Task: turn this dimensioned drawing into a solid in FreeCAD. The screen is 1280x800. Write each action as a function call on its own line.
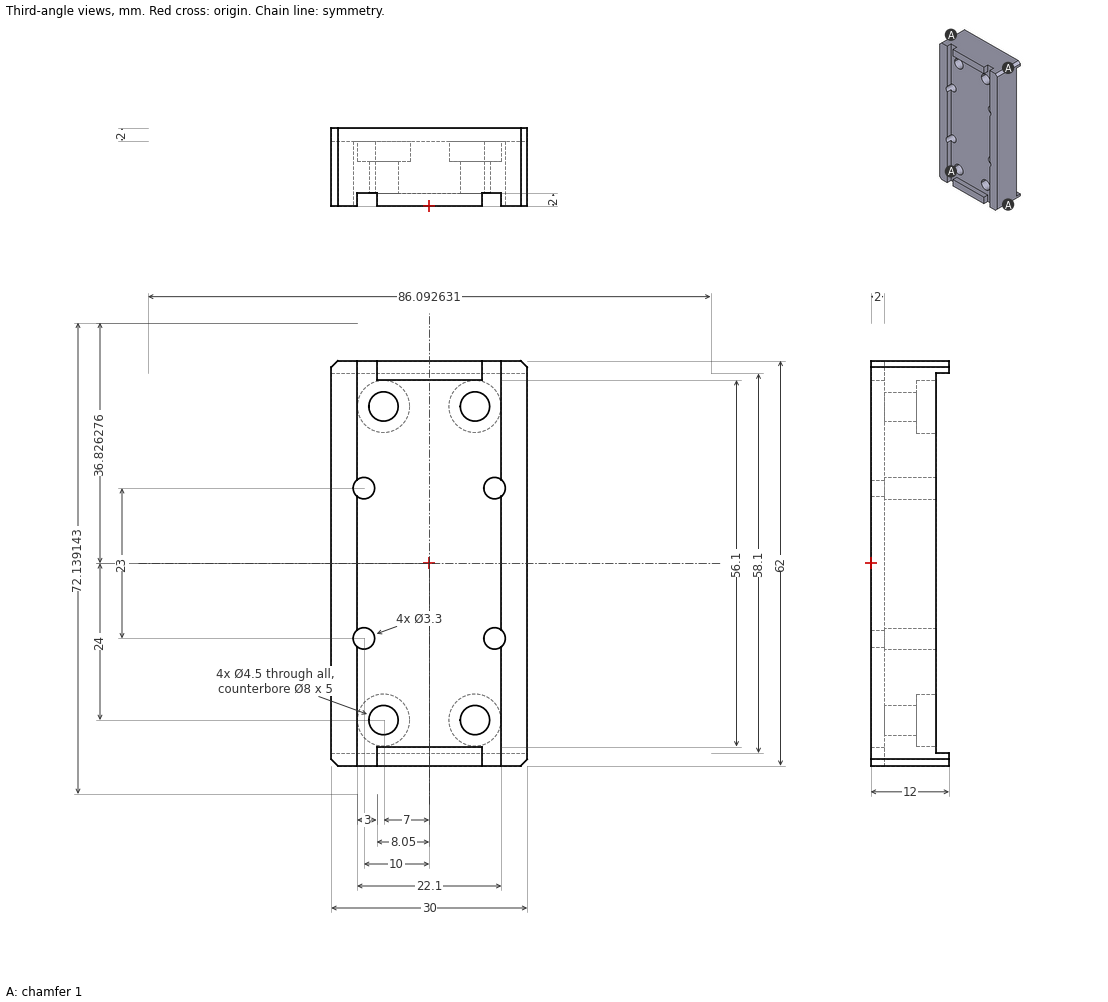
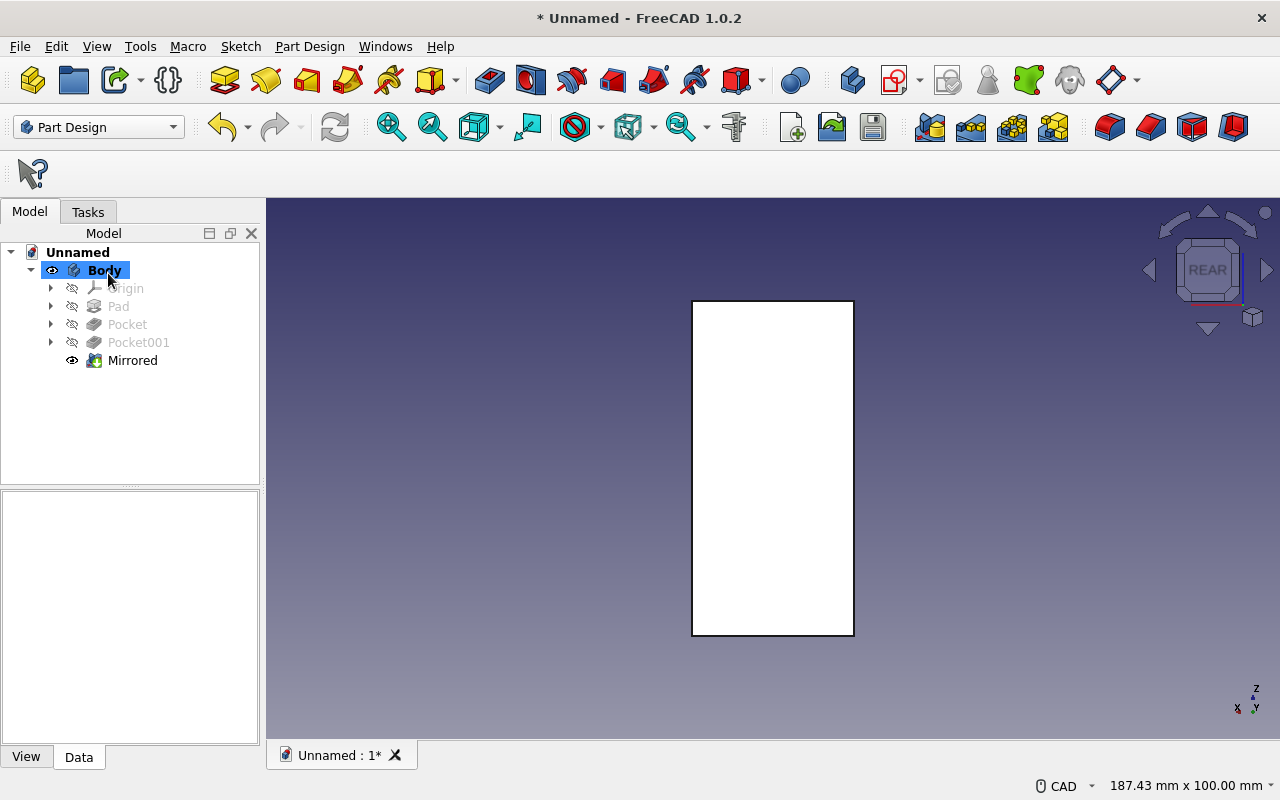
click(773, 420)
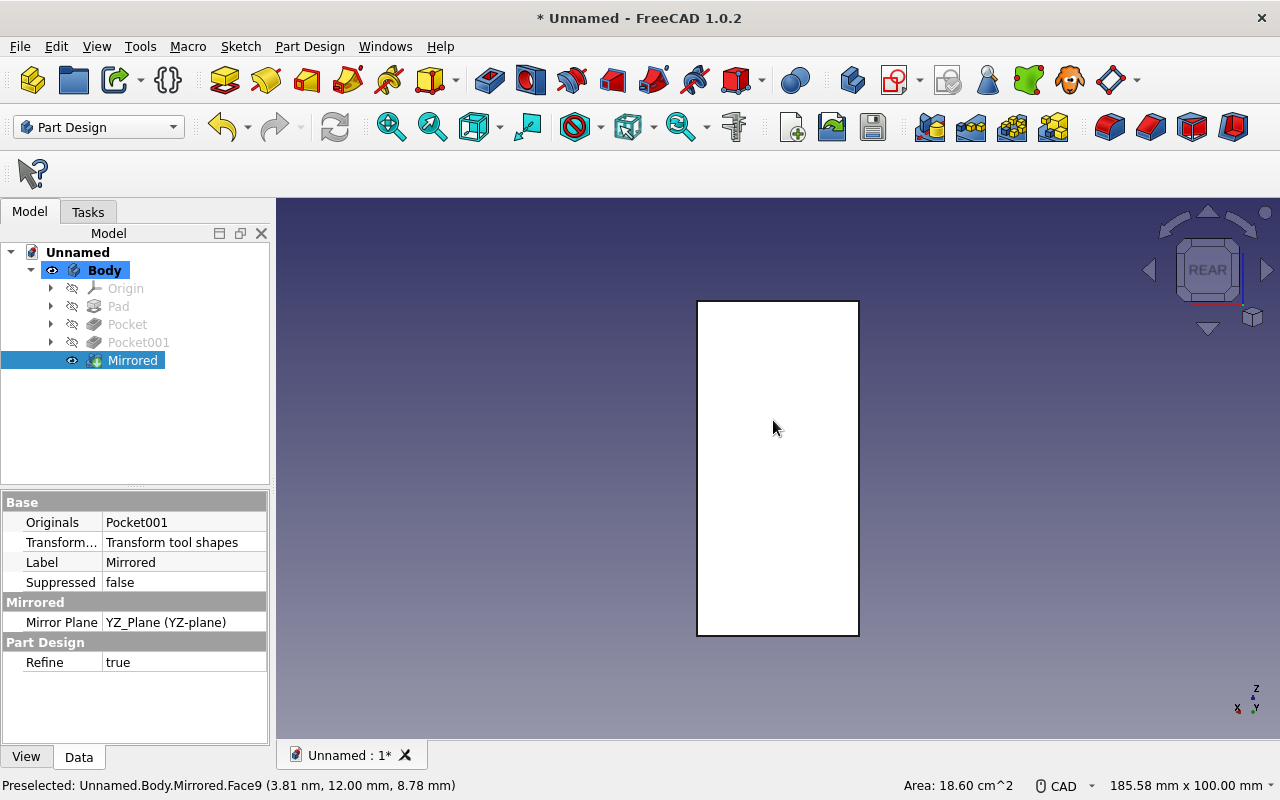
click(894, 80)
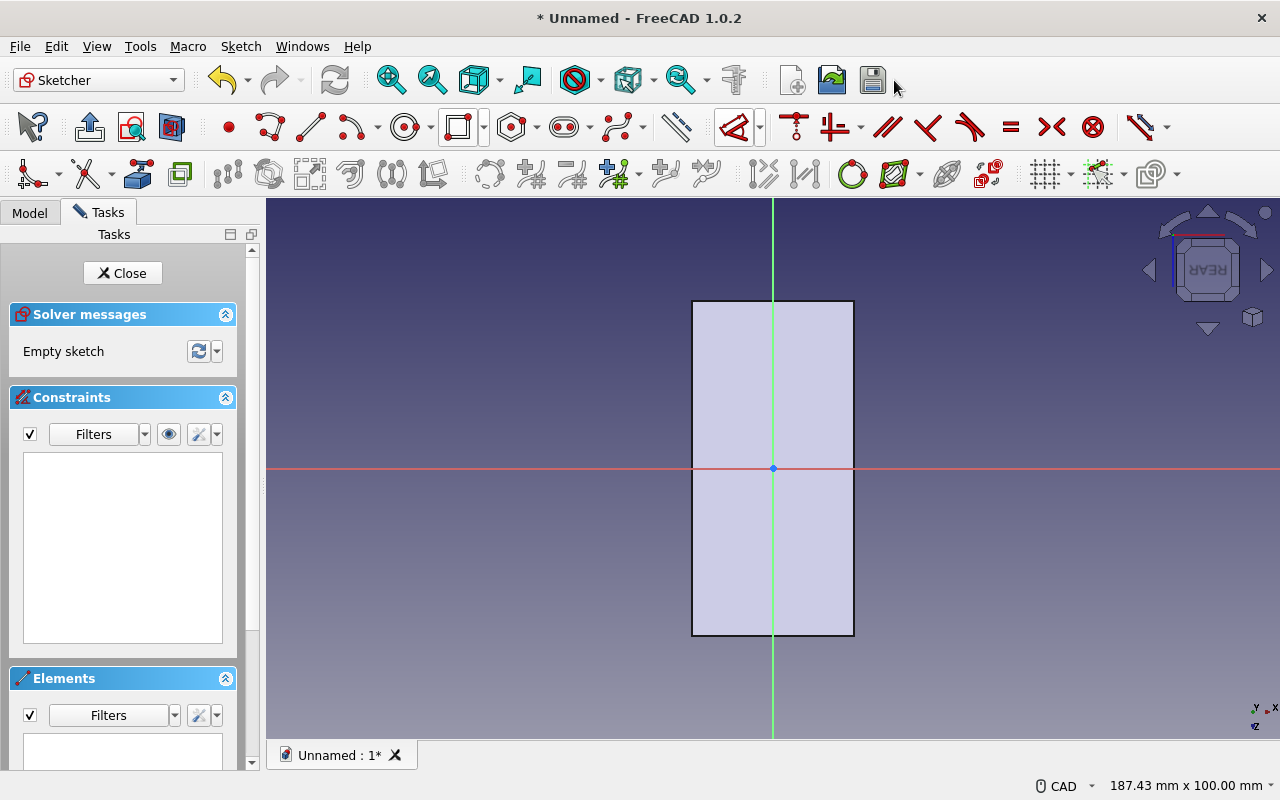
click(484, 128)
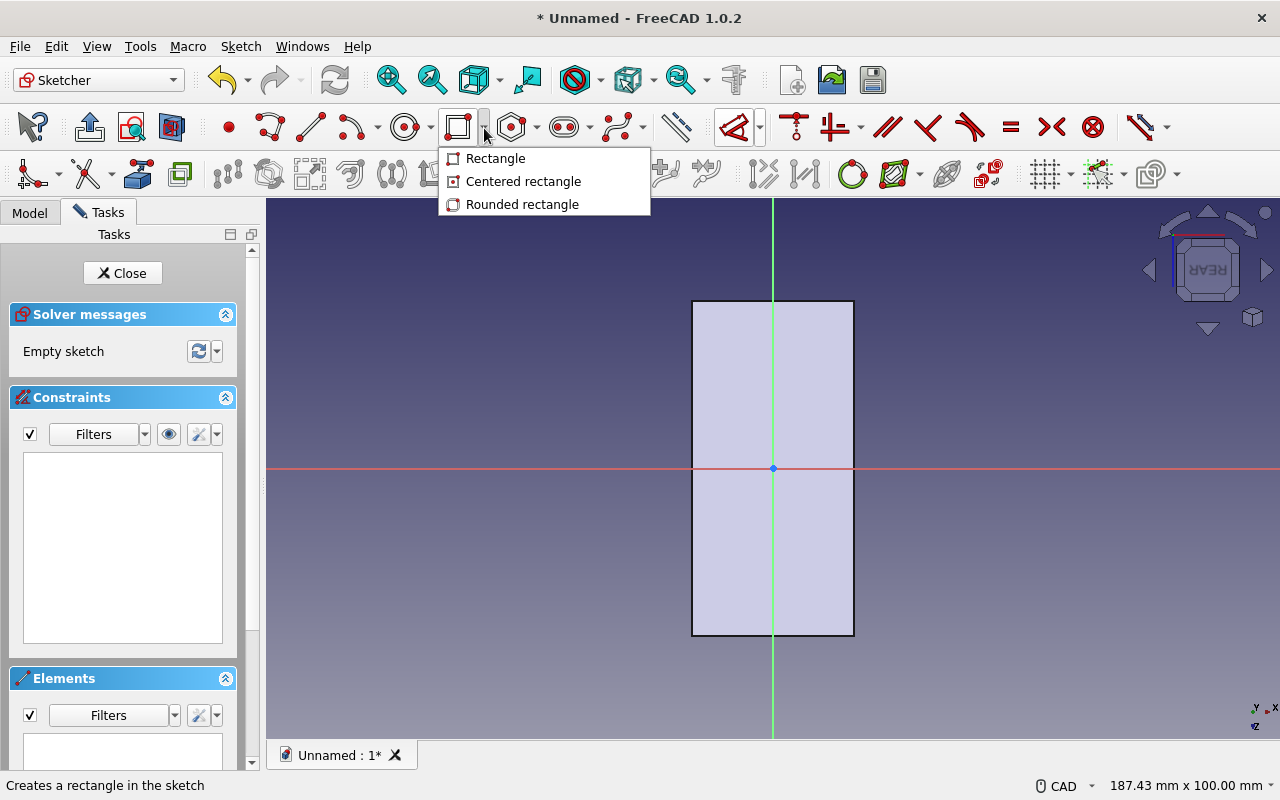
click(544, 182)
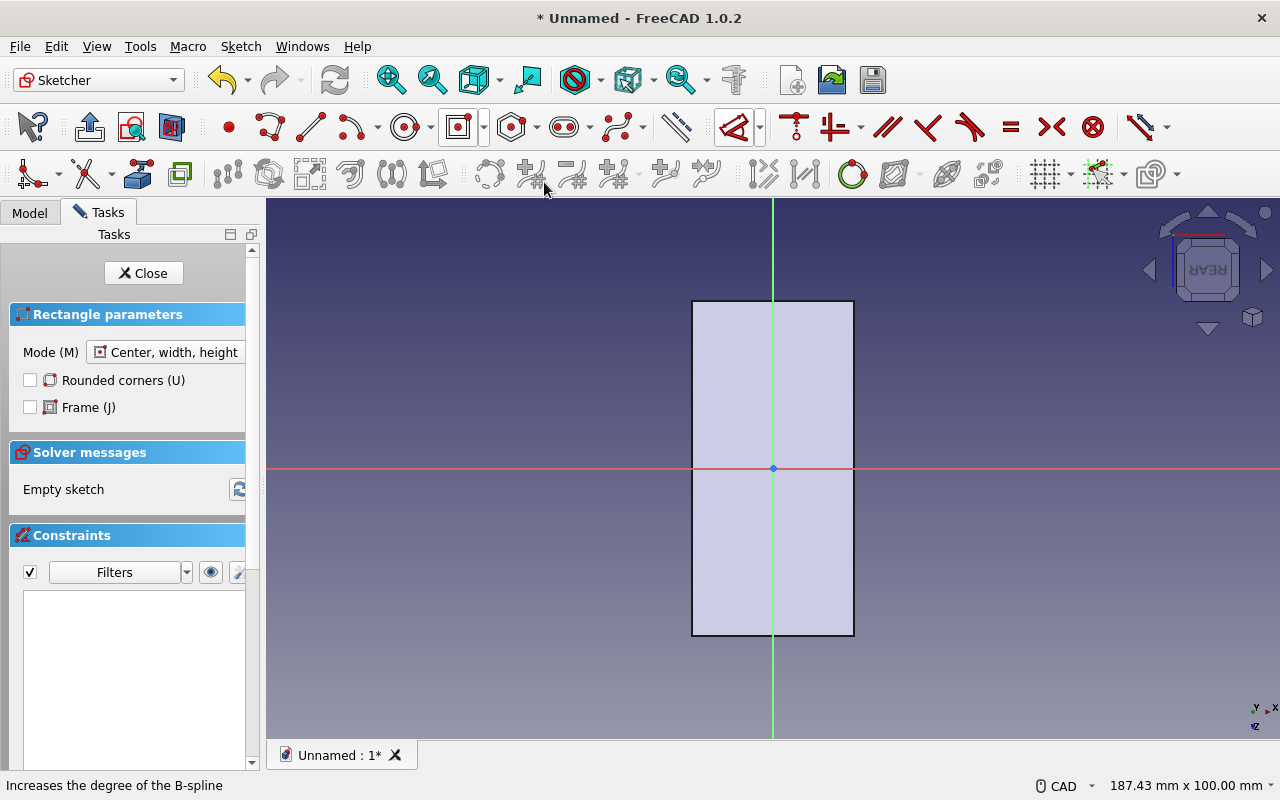
click(773, 469)
click(1006, 311)
key(Escape)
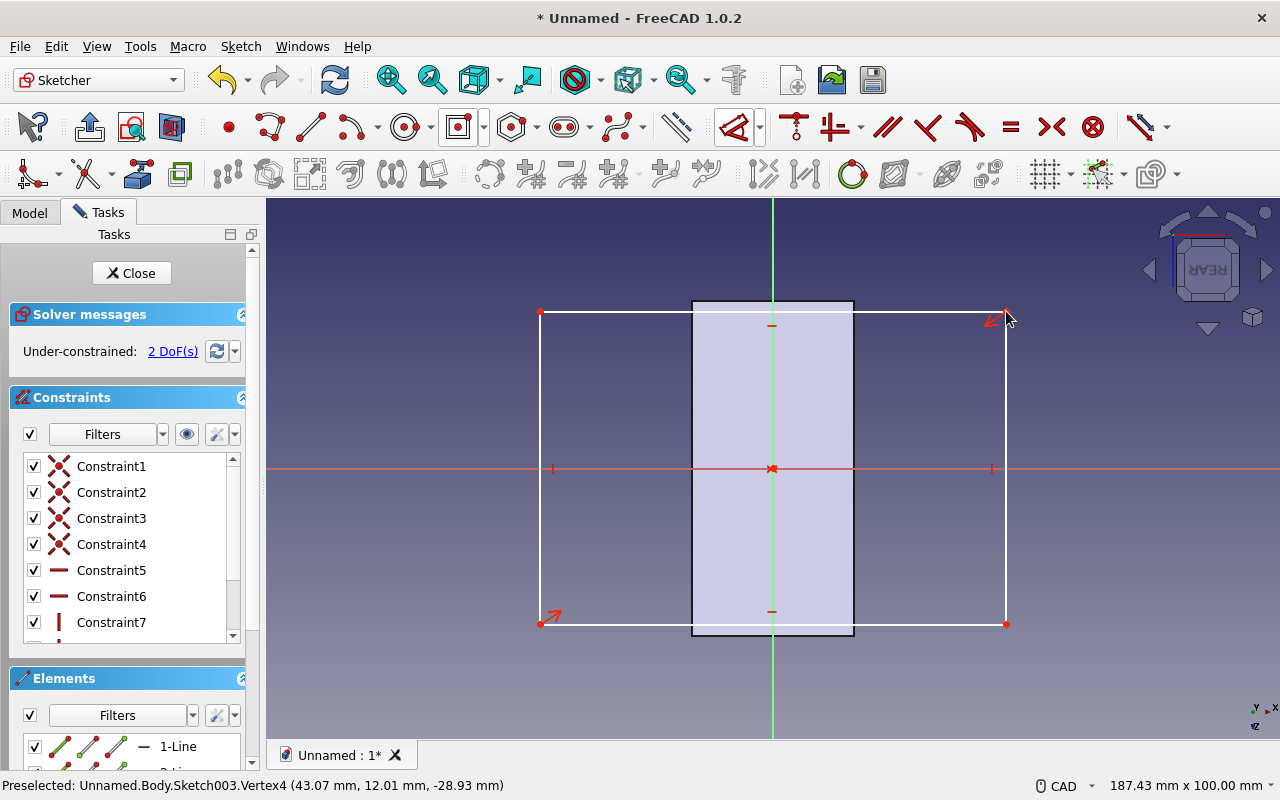
click(1006, 531)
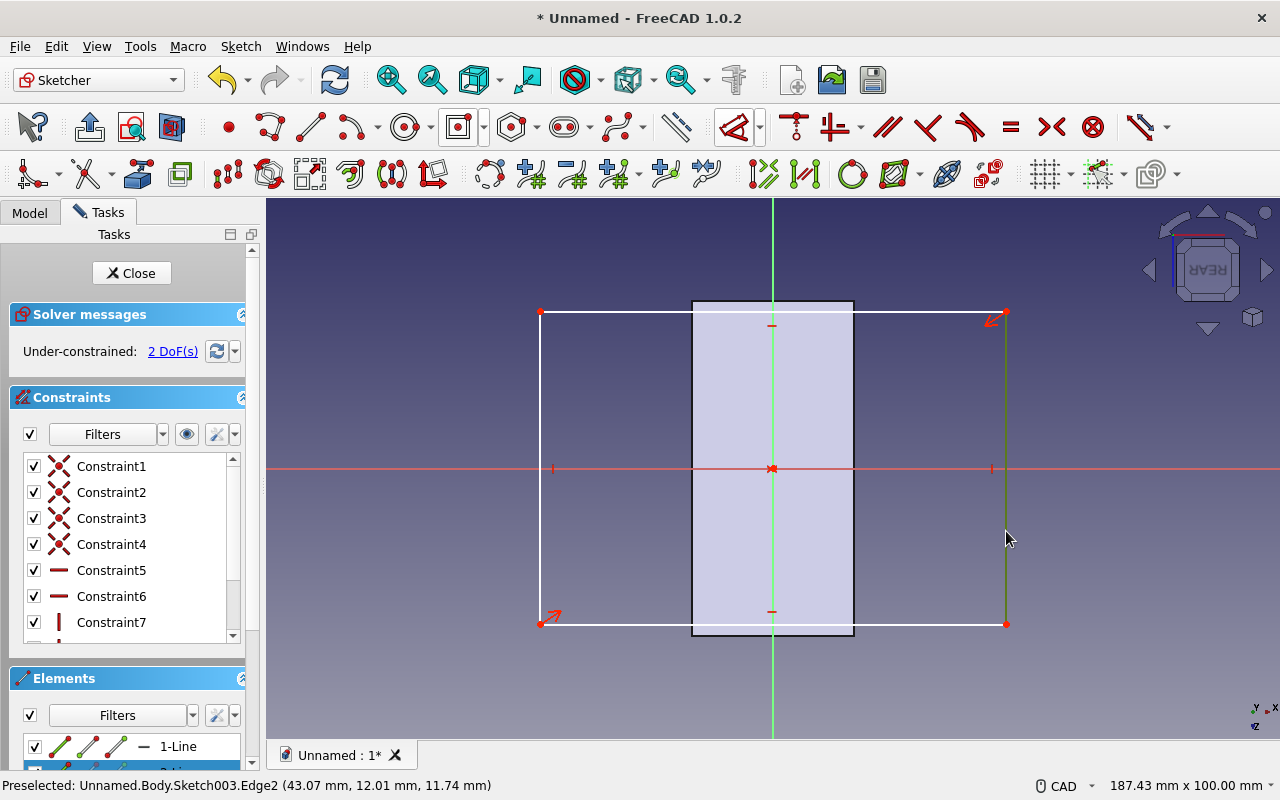
click(760, 128)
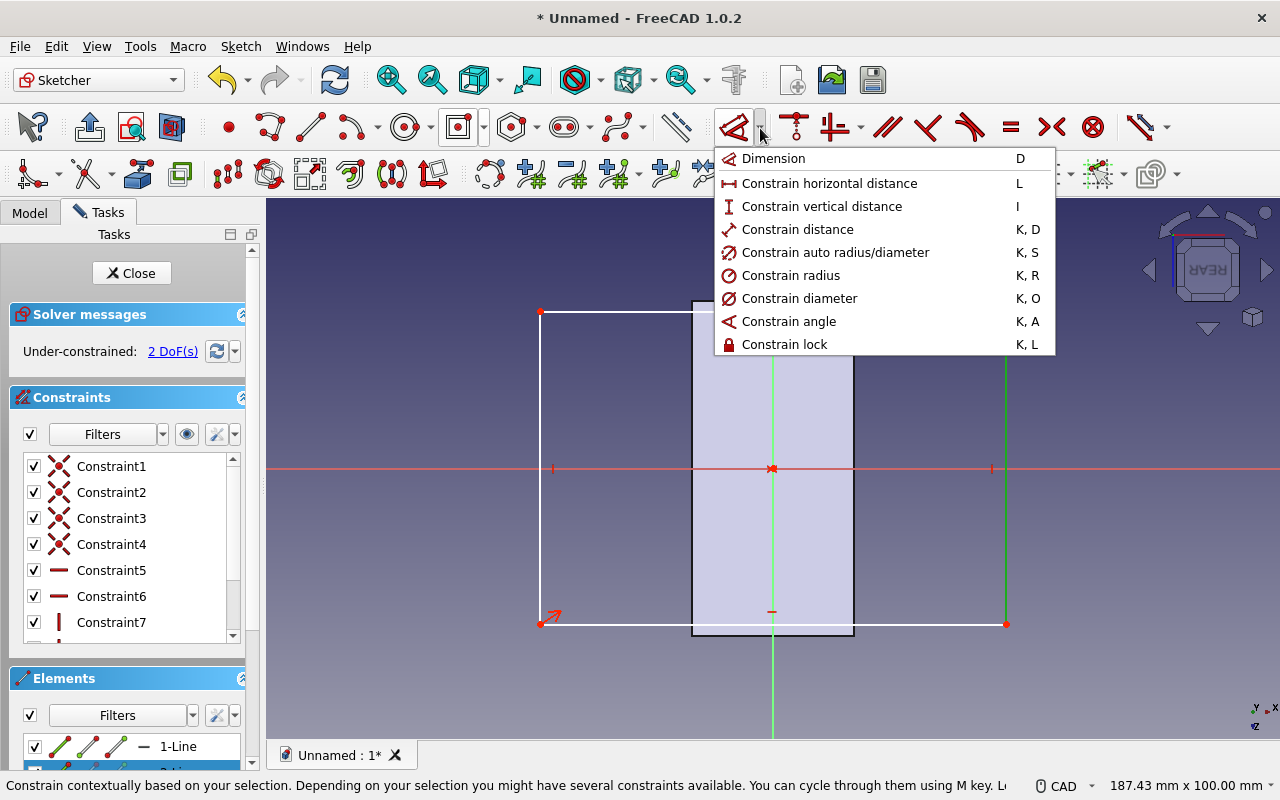
click(885, 206)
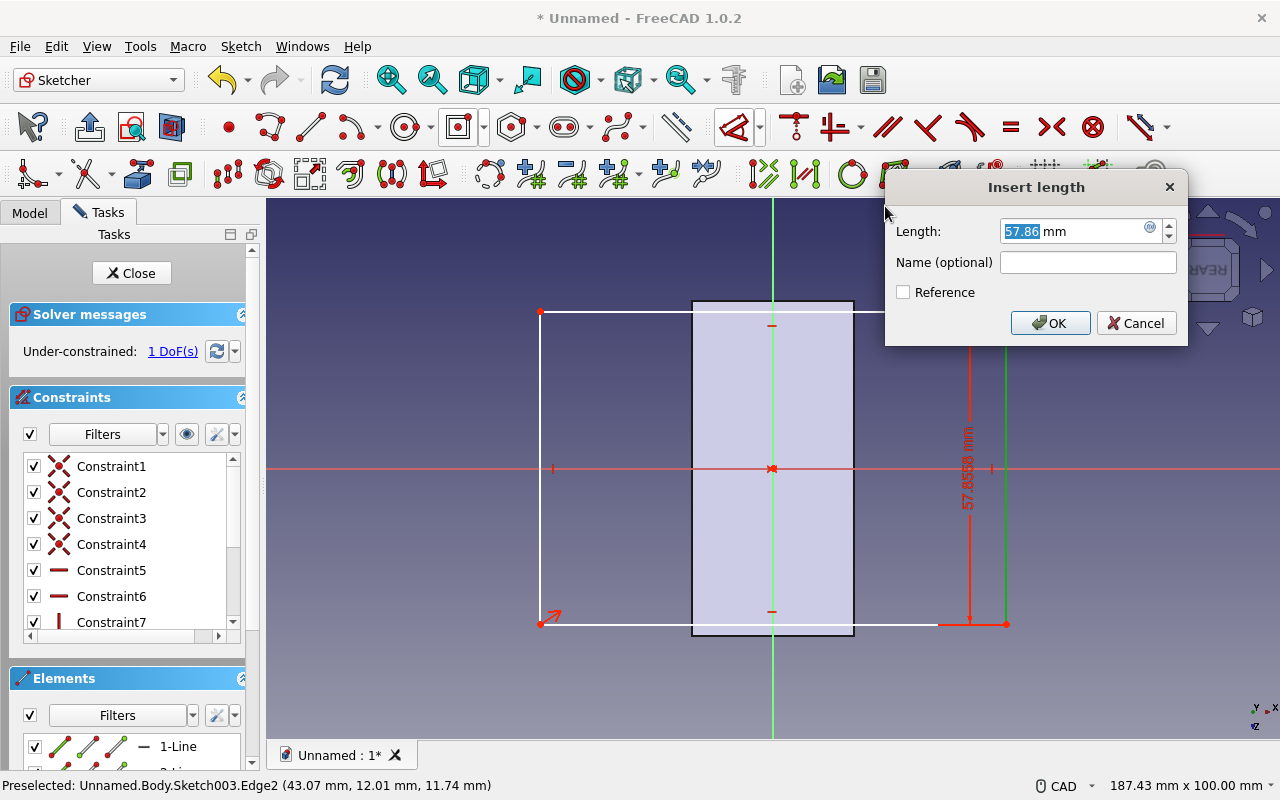
text(58.1)
key(Return)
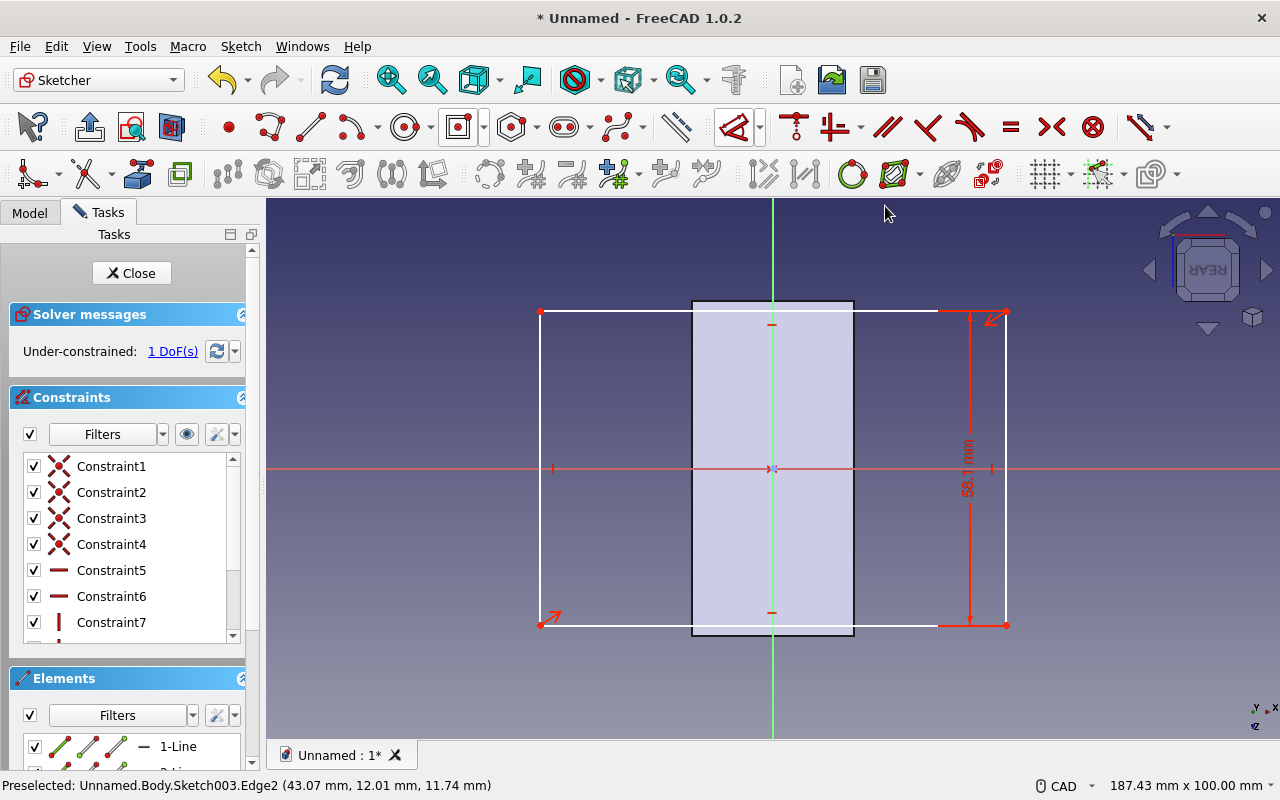
click(680, 626)